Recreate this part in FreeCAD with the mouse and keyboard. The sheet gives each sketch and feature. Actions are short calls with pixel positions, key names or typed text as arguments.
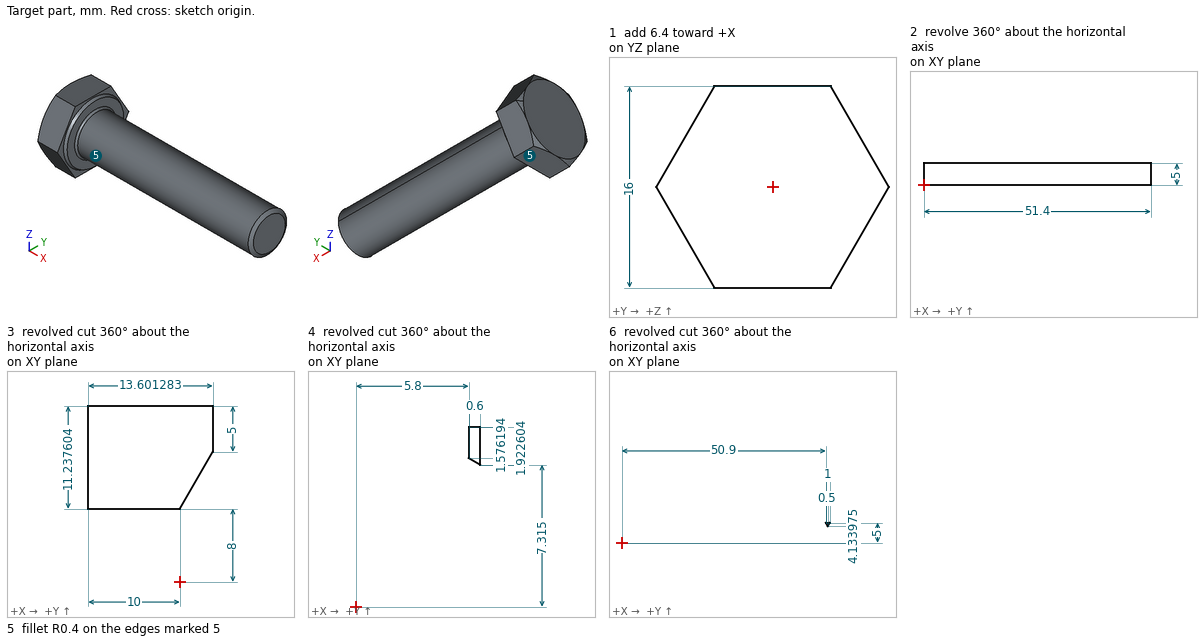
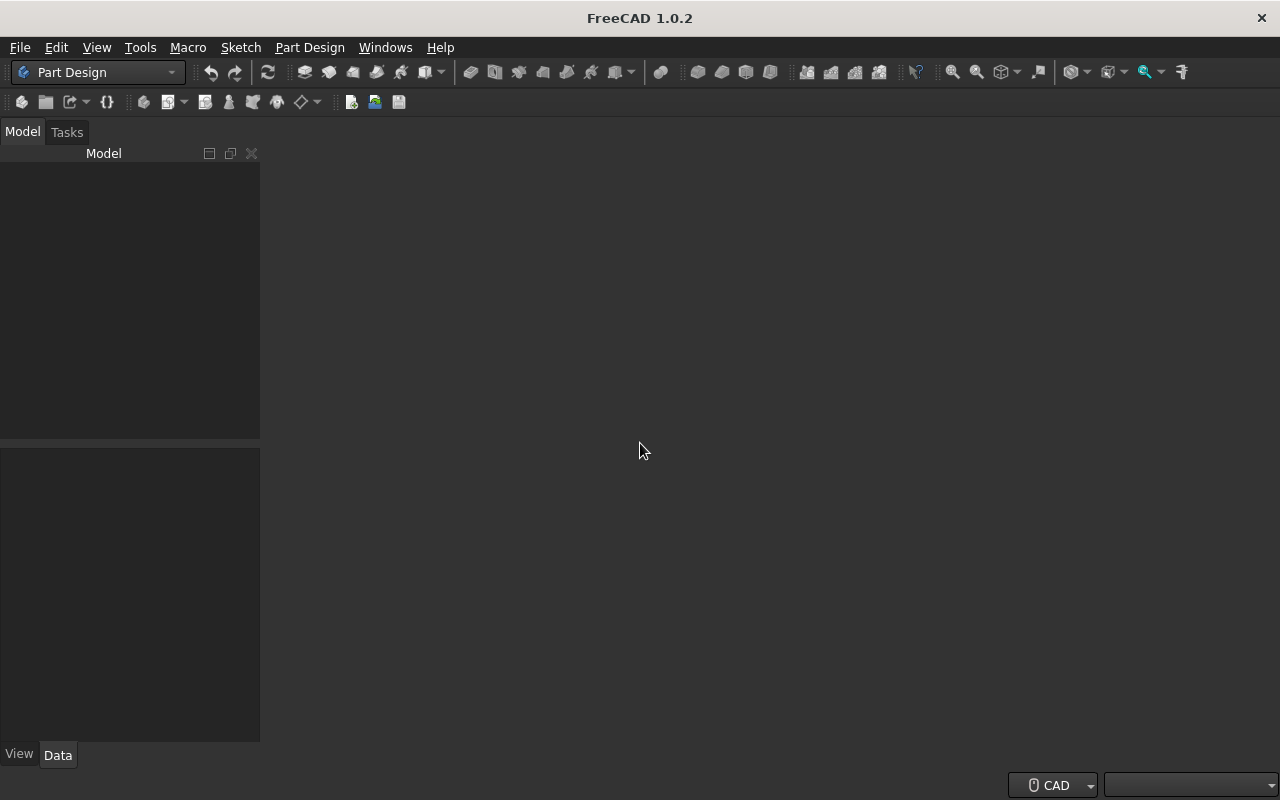
click(352, 102)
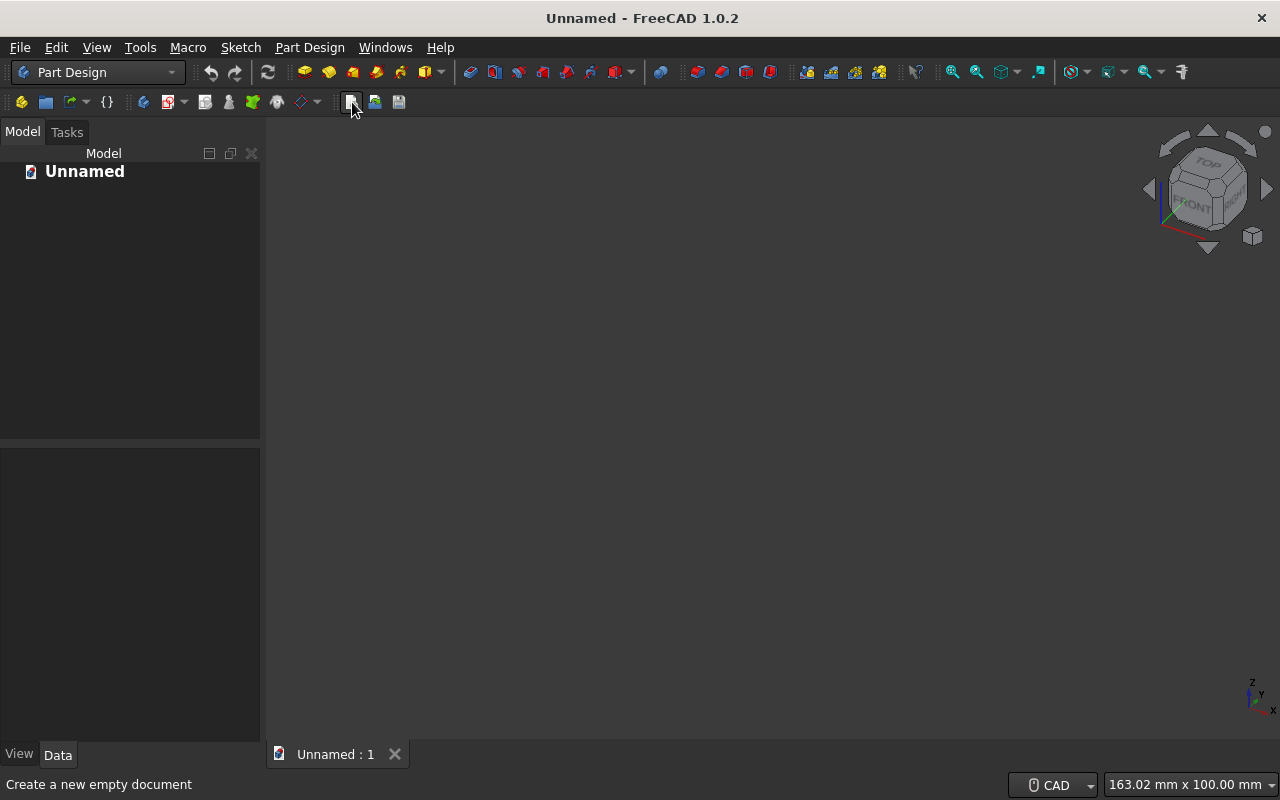
click(168, 102)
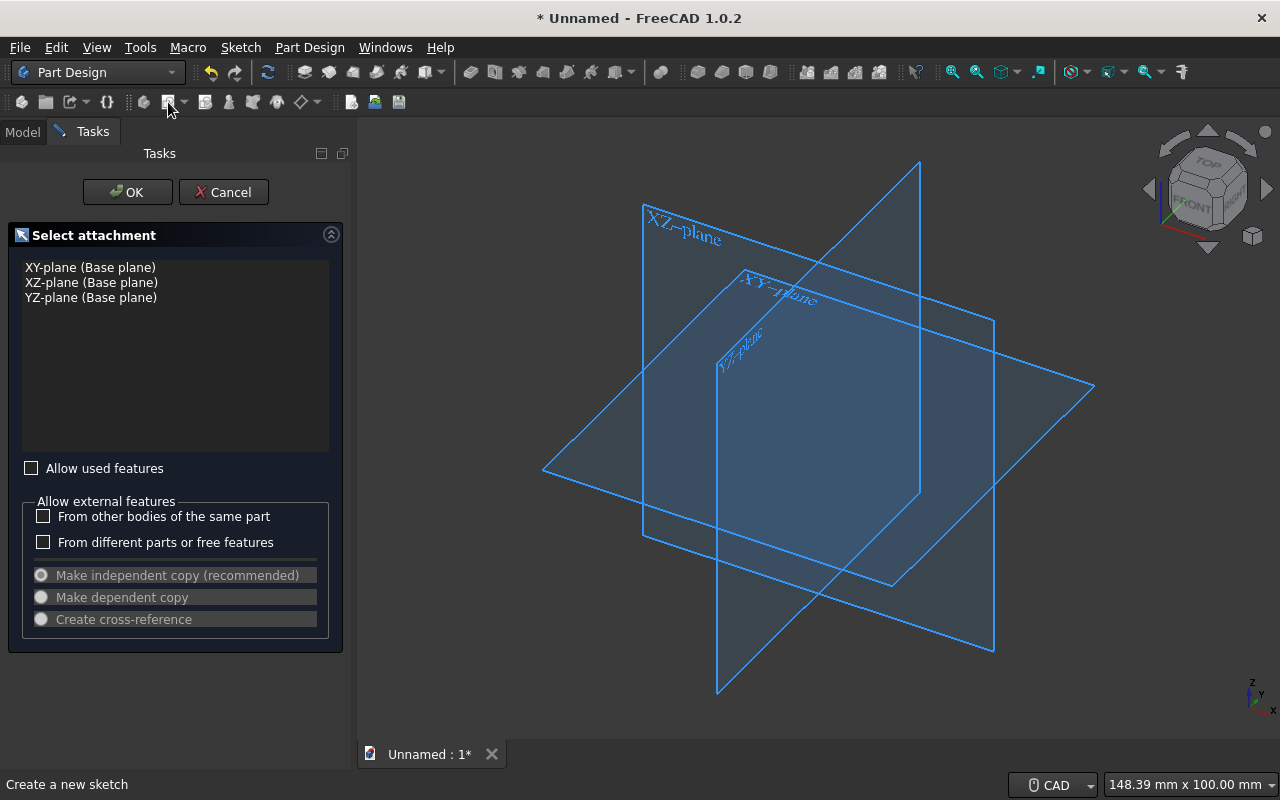
click(82, 298)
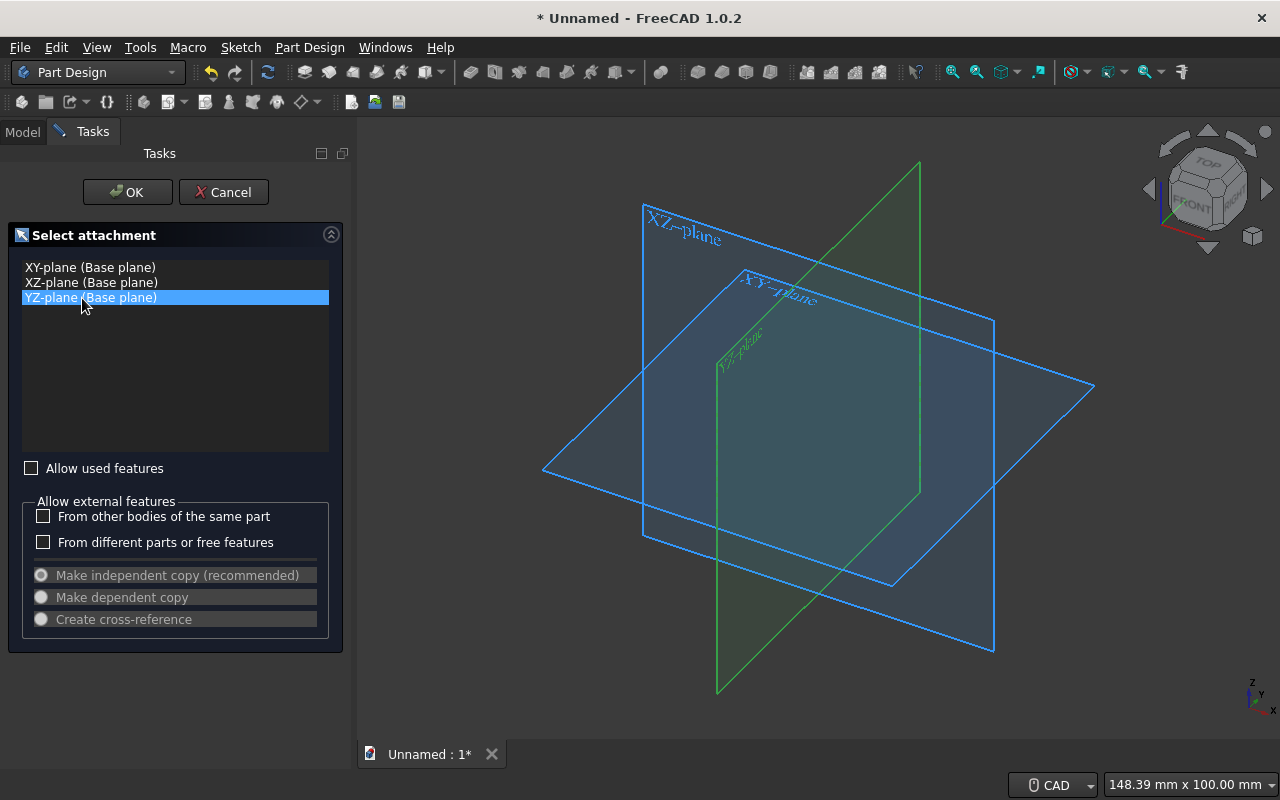
click(128, 192)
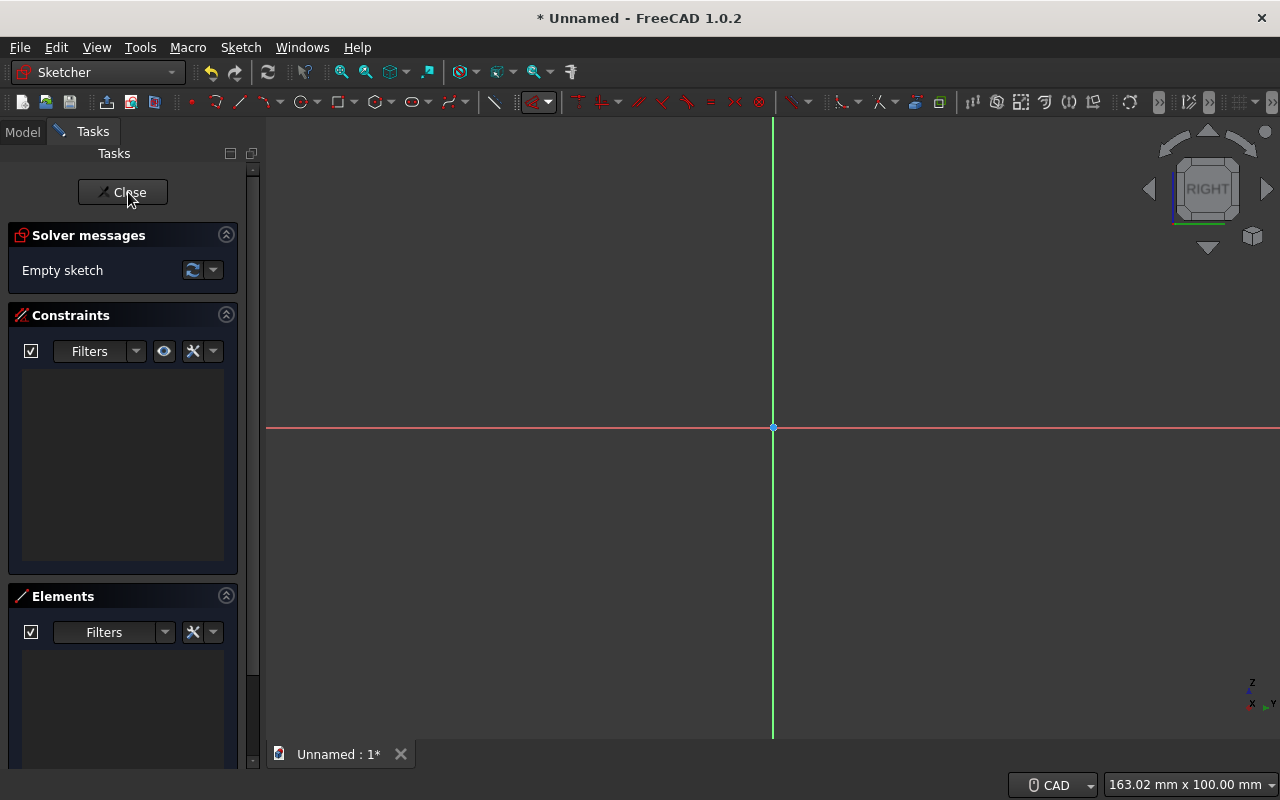
scroll(795, 428, up, 7)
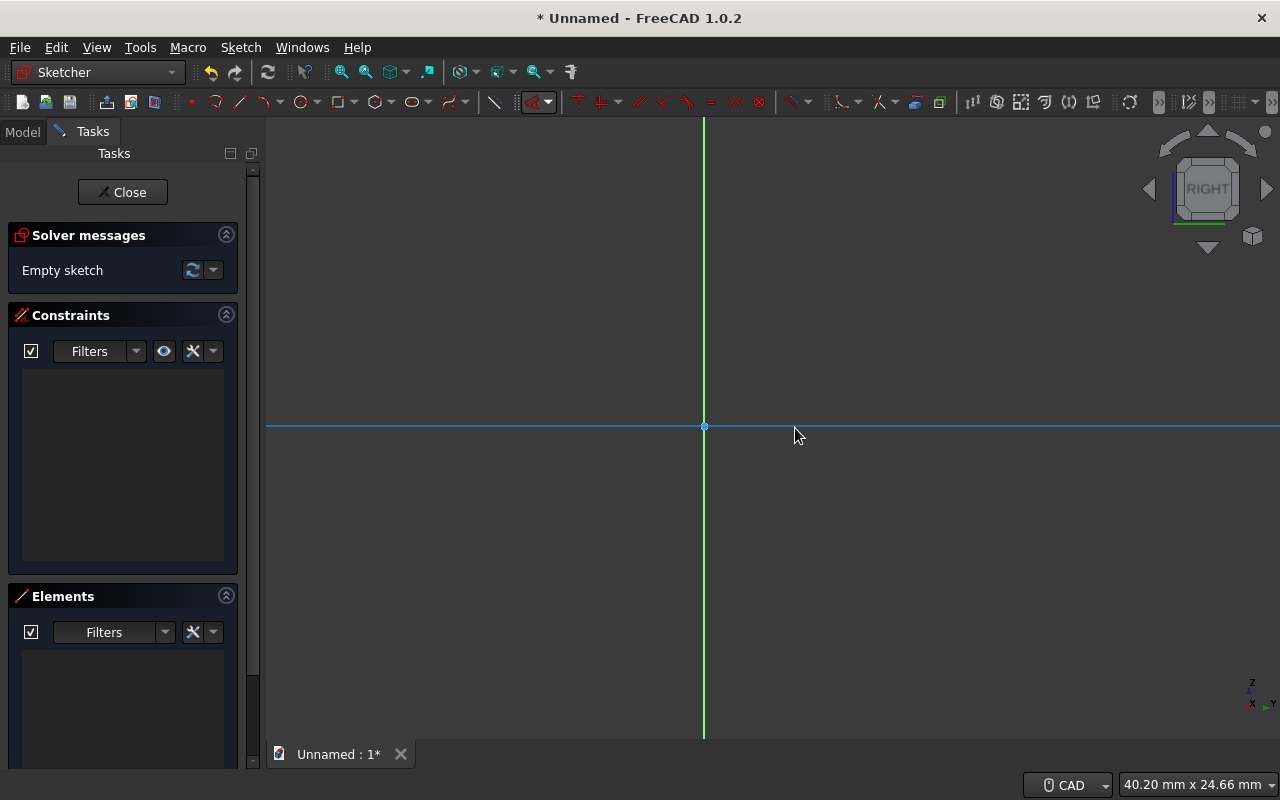
click(376, 102)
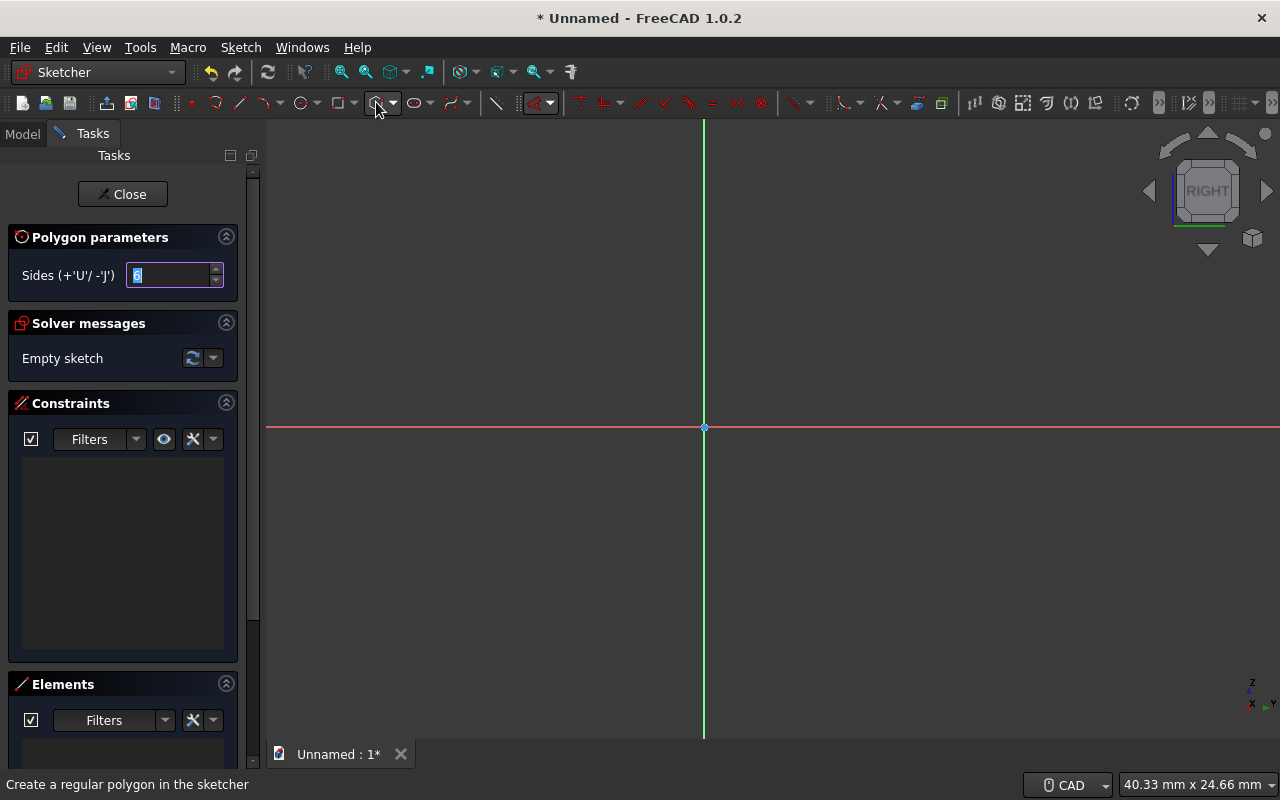
click(704, 427)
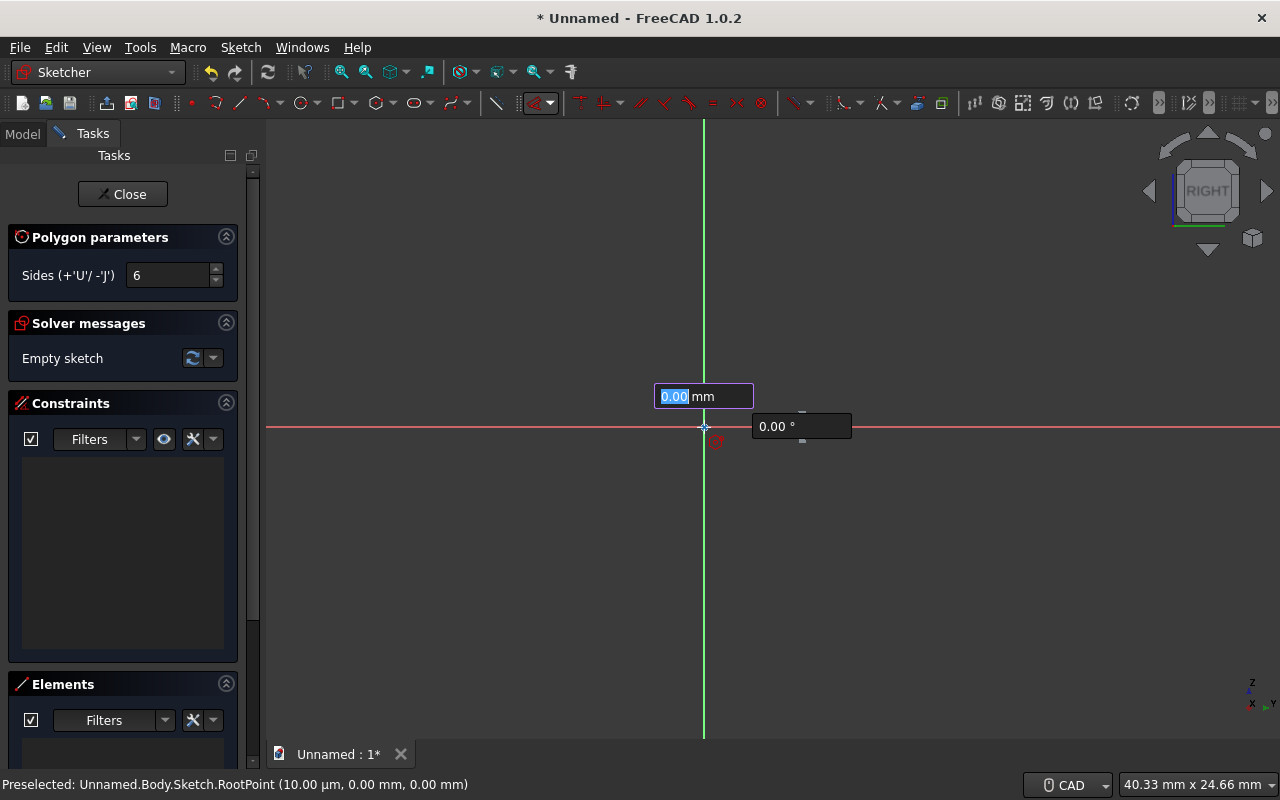
click(937, 427)
right_click(937, 427)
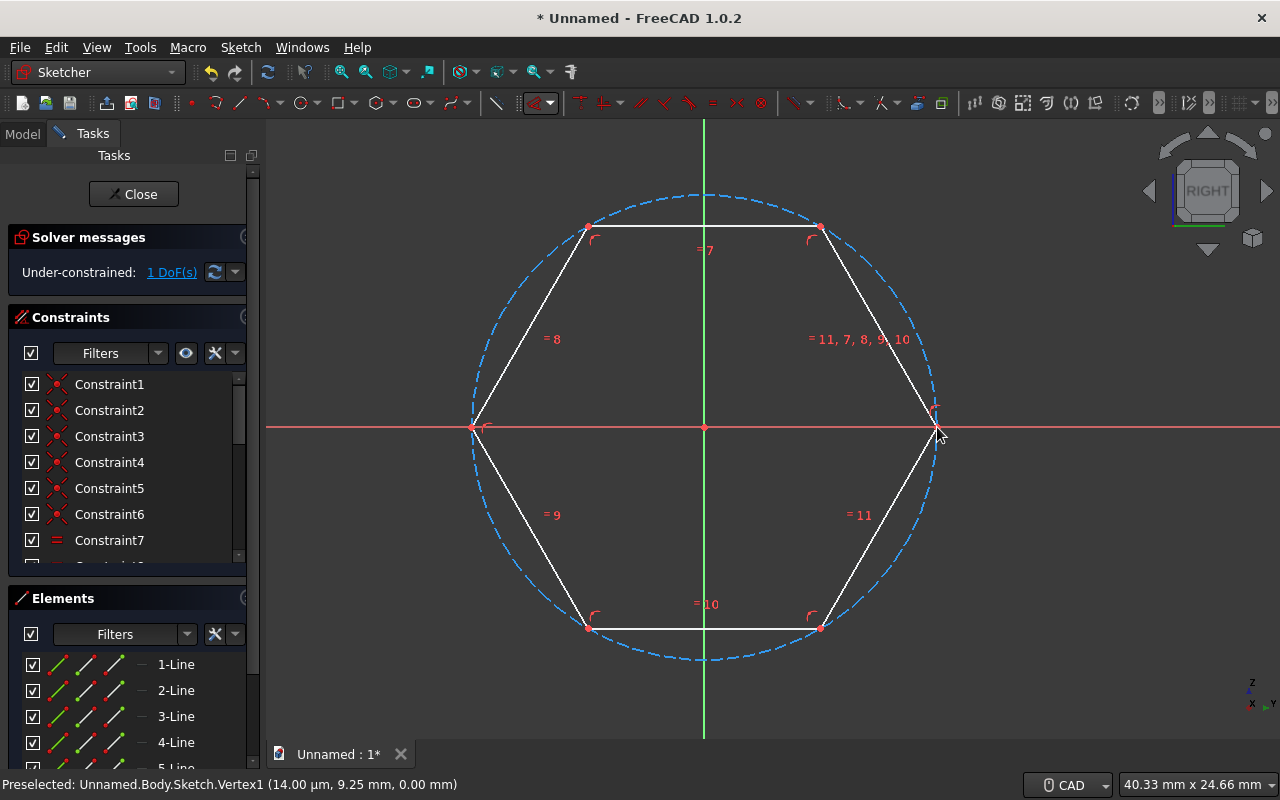
click(534, 104)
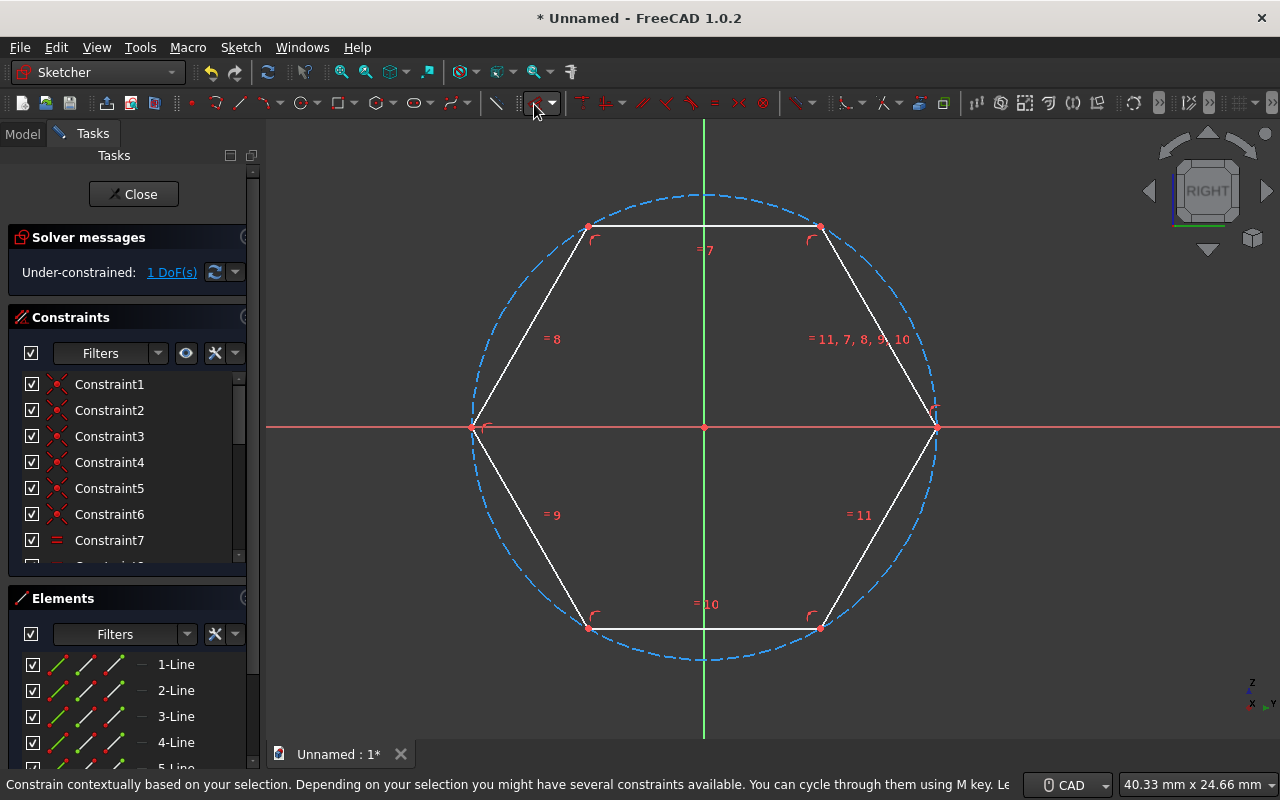
click(588, 629)